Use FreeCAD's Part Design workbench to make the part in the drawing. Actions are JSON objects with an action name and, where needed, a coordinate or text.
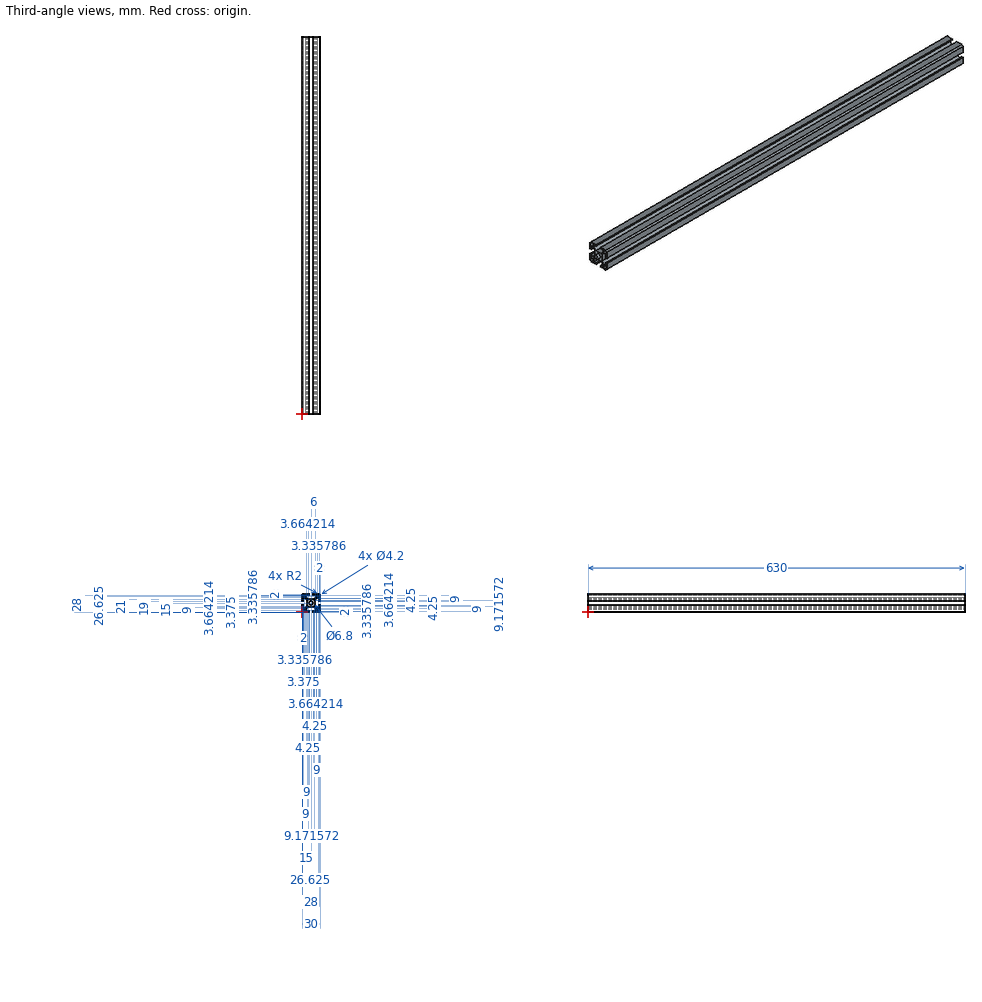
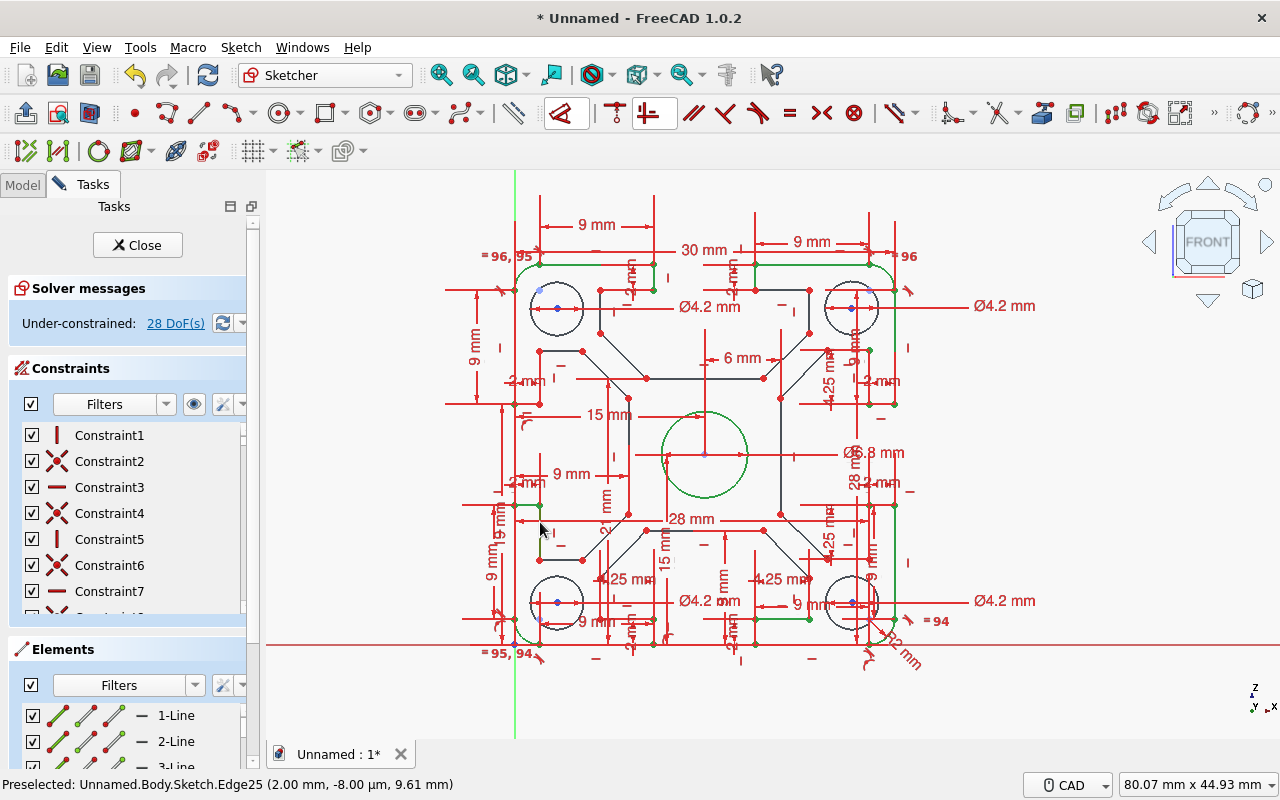
{"action": "left_click", "coordinate": [584, 114]}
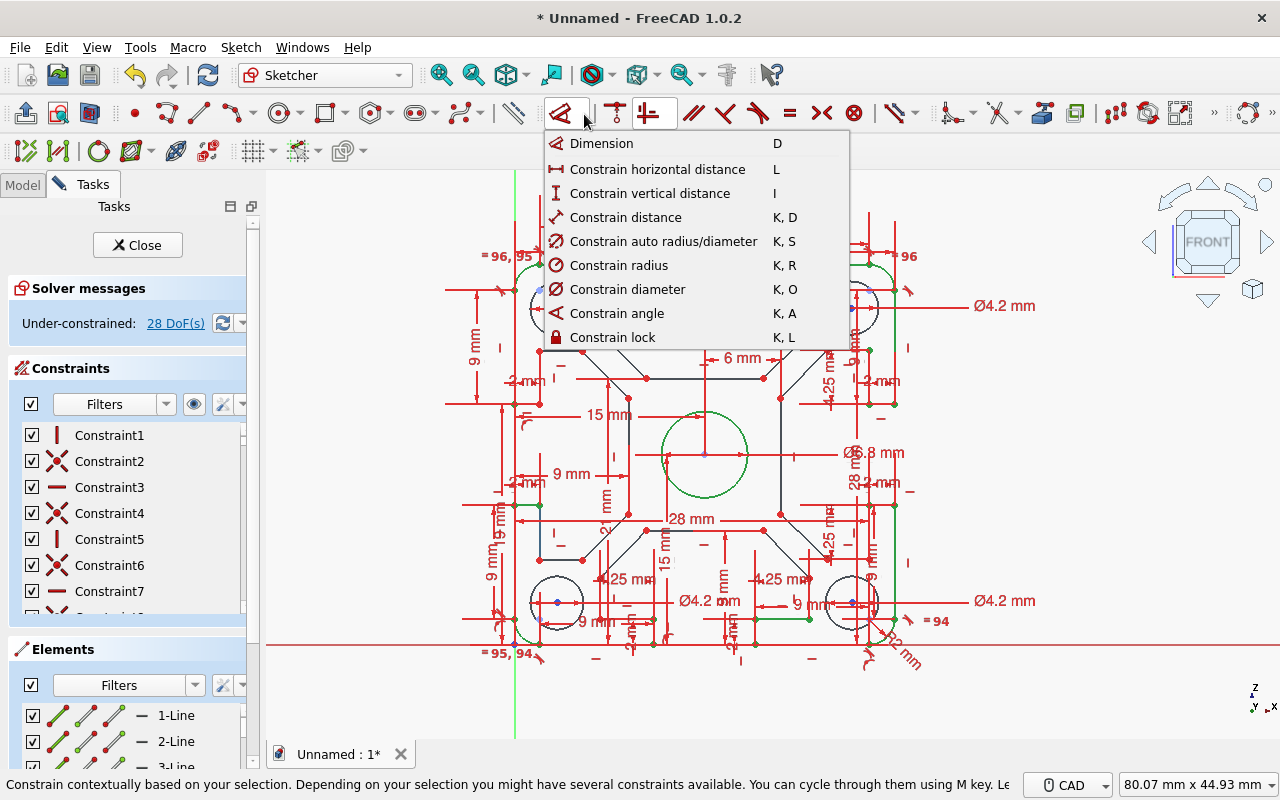
{"action": "left_click", "coordinate": [697, 193]}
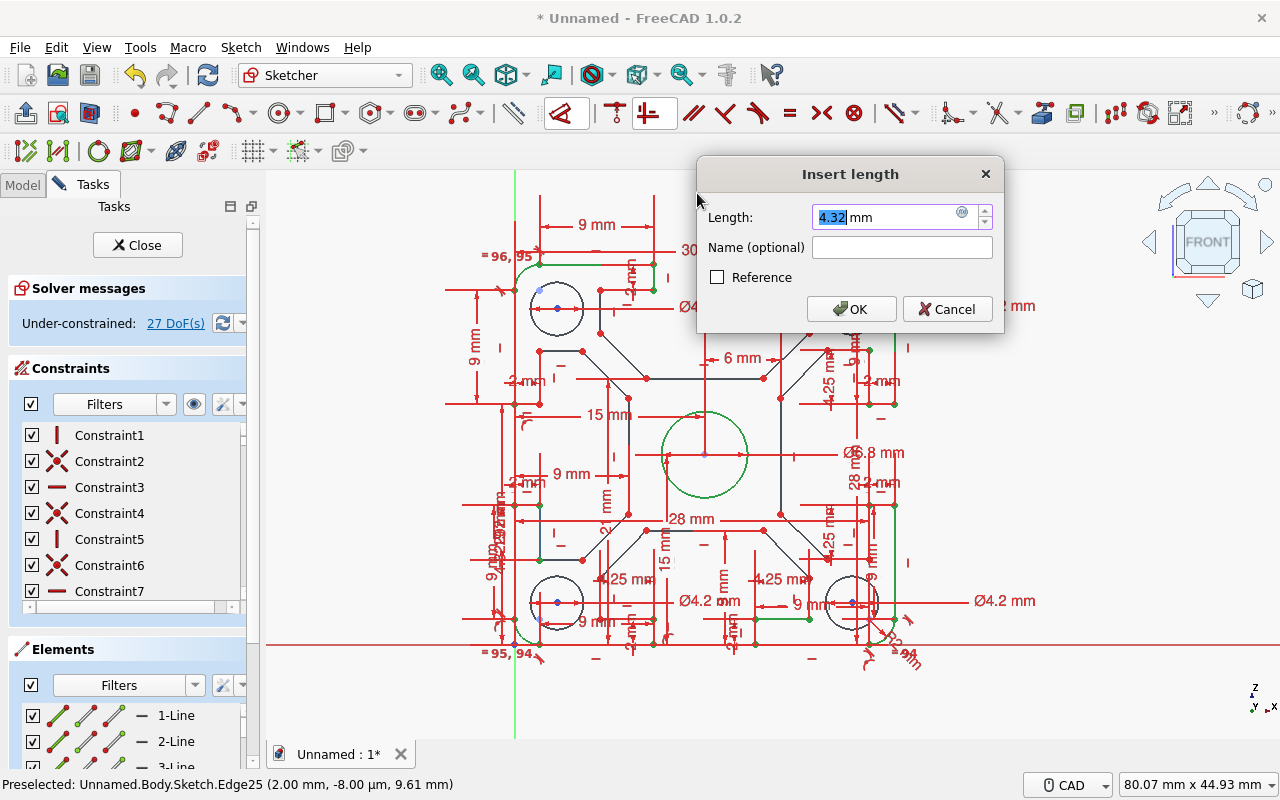
{"action": "type", "text": "4.25"}
{"action": "key", "text": "Return"}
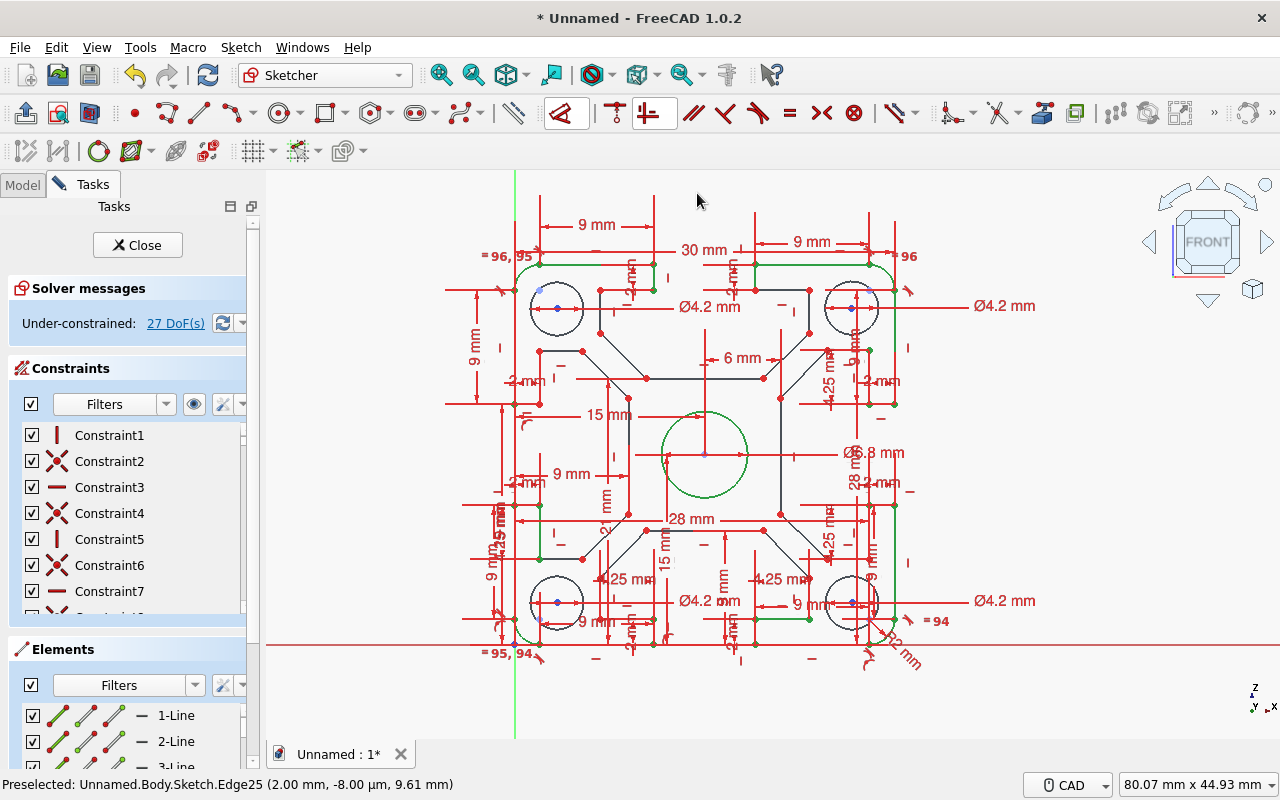
{"action": "left_click", "coordinate": [540, 367]}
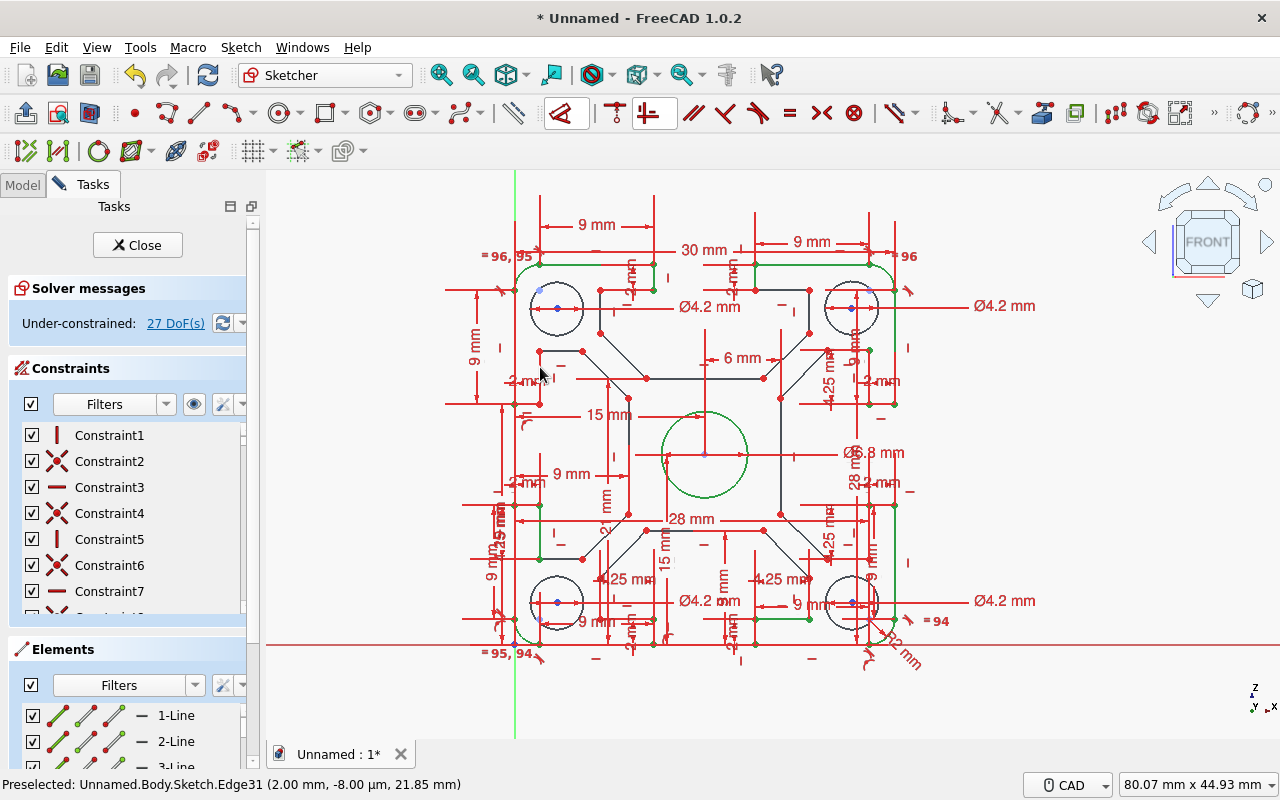
{"action": "key", "text": "i"}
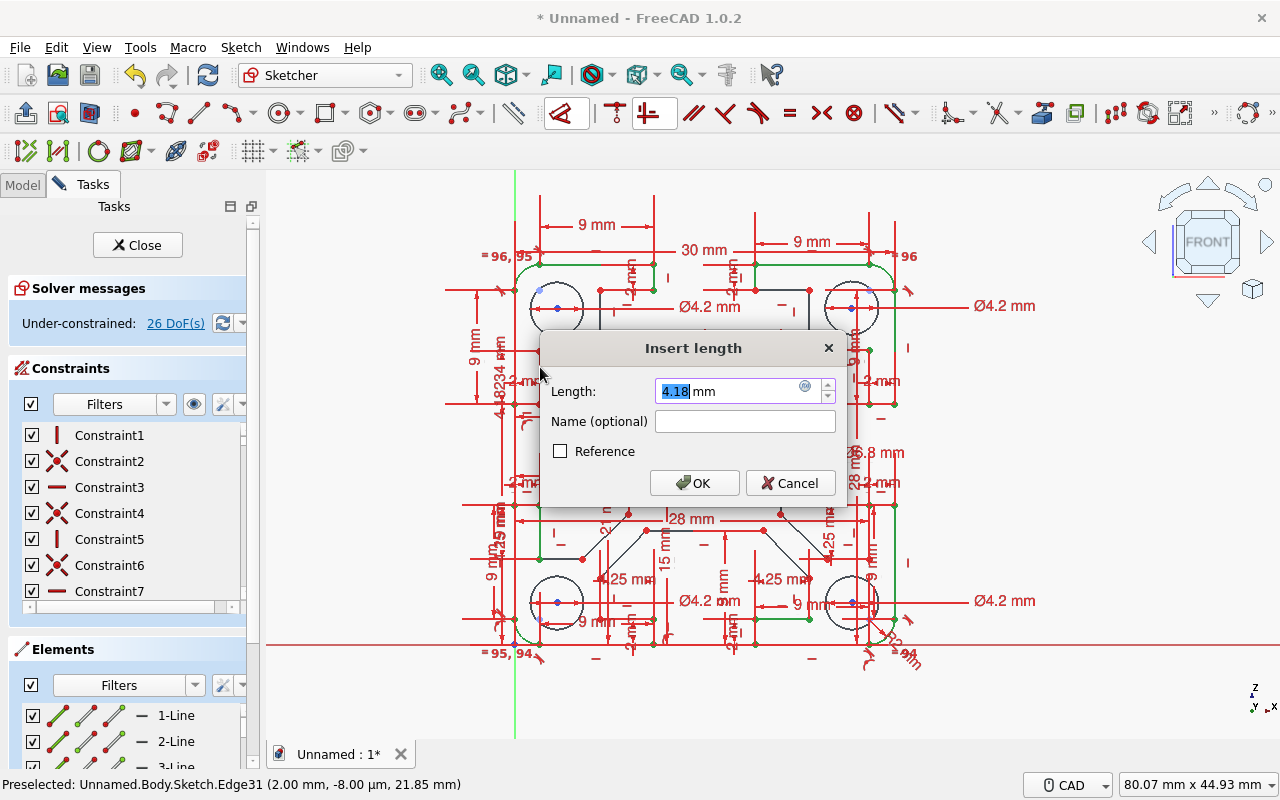
{"action": "type", "text": "4.25"}
{"action": "key", "text": "Return"}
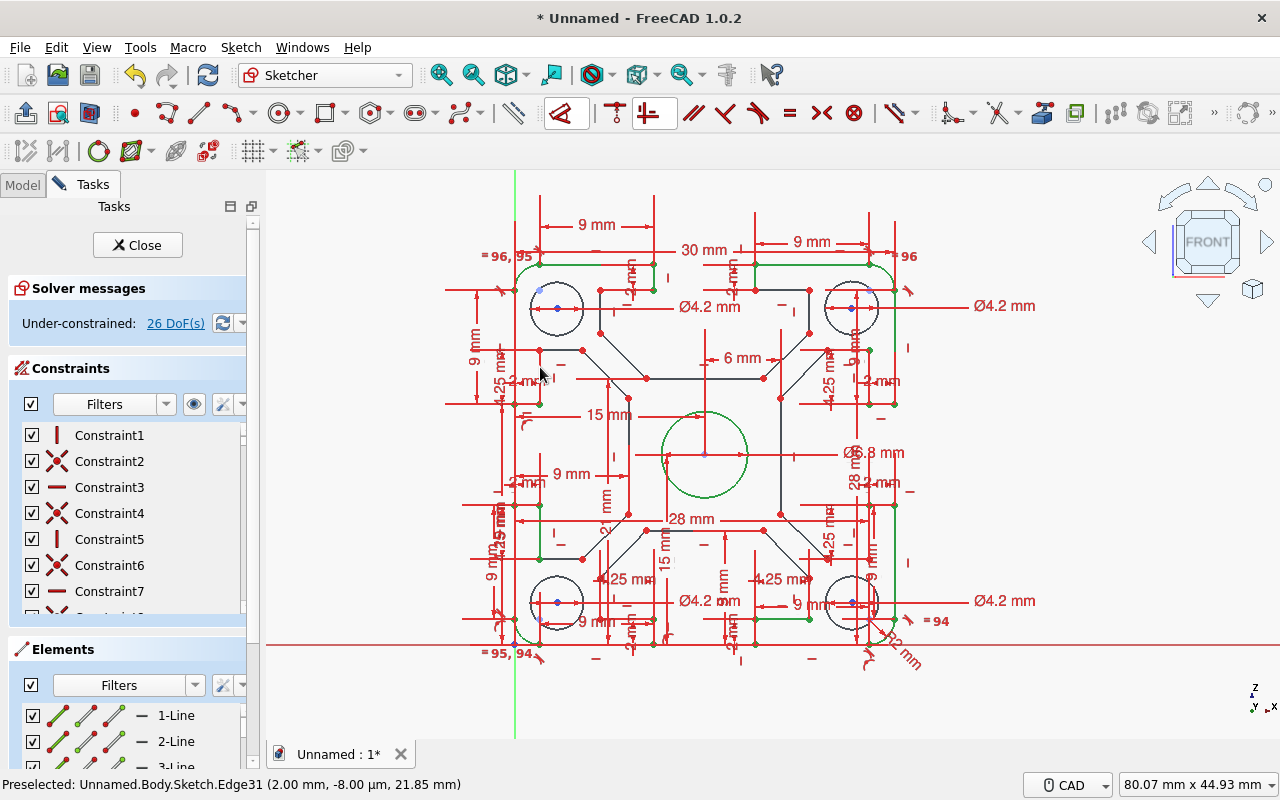
{"action": "left_click", "coordinate": [616, 290]}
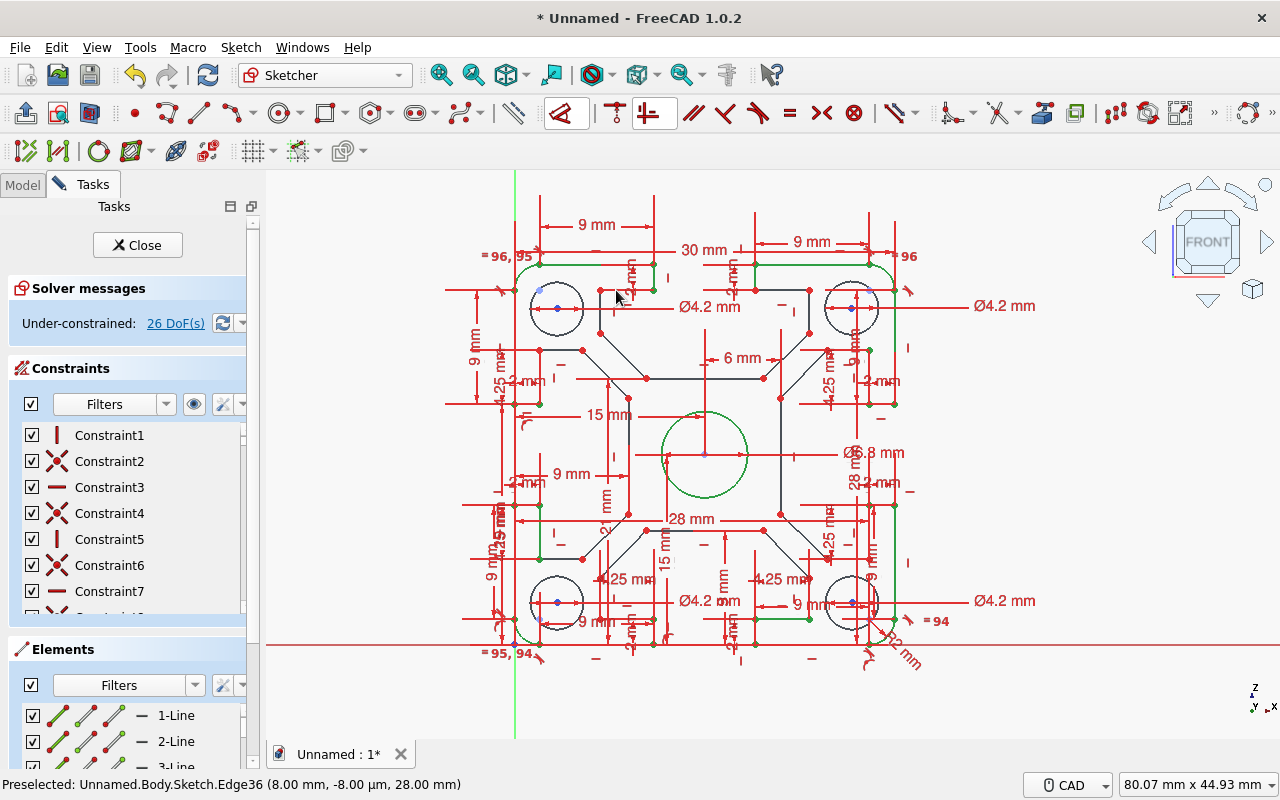
{"action": "left_click", "coordinate": [584, 114]}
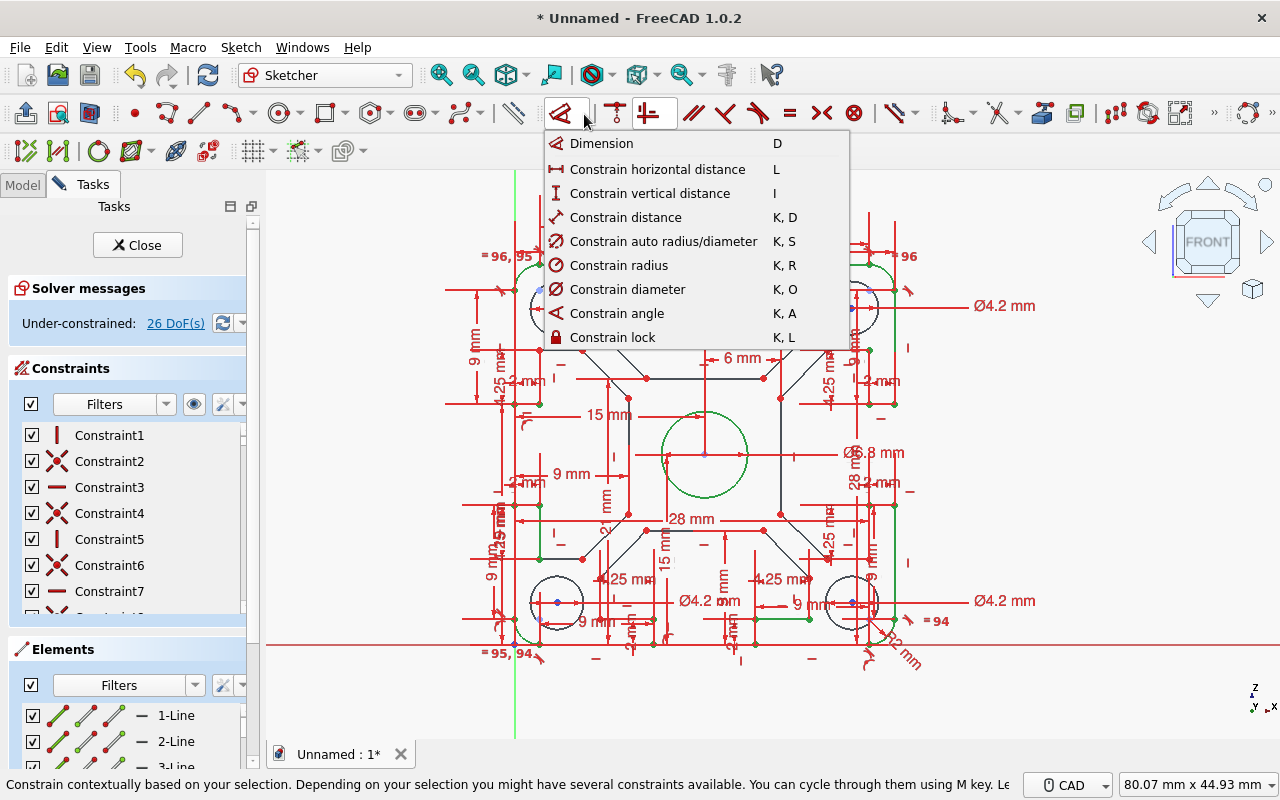
{"action": "left_click", "coordinate": [697, 169]}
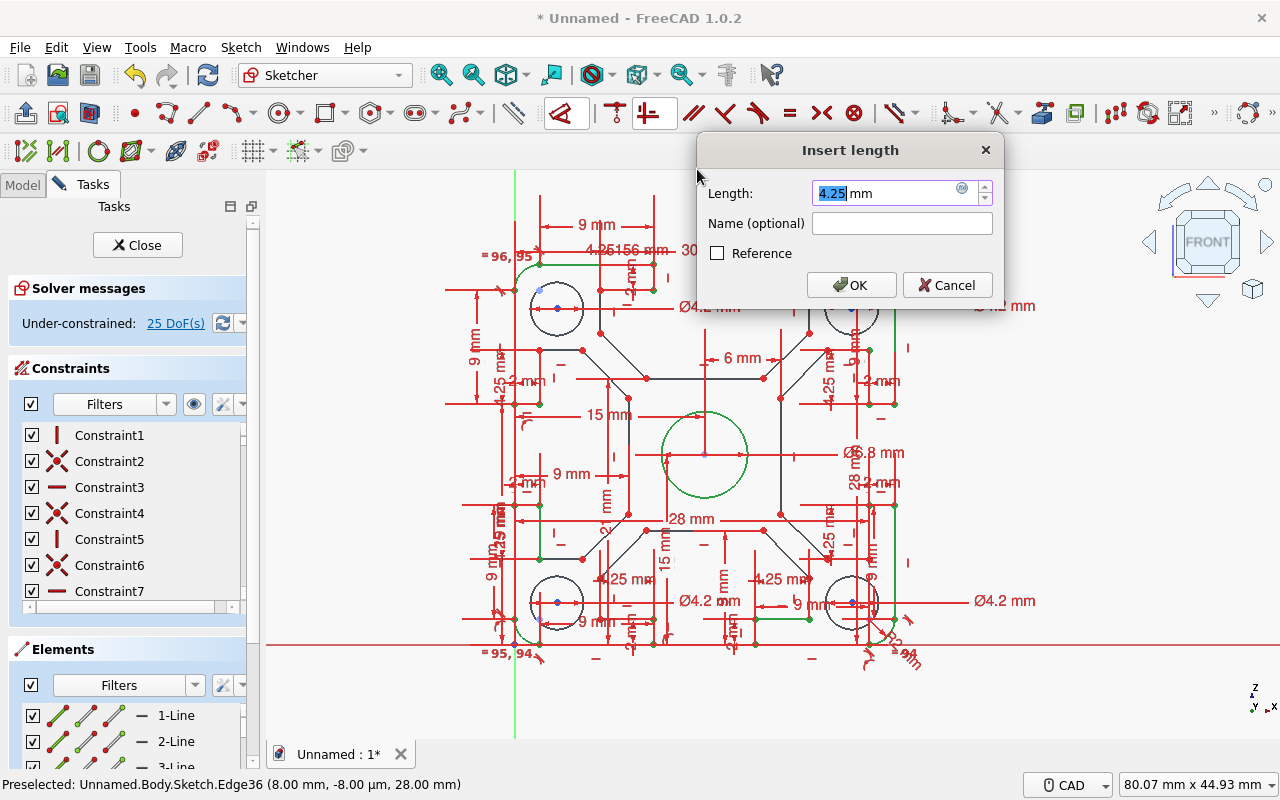
{"action": "type", "text": "4.25"}
{"action": "key", "text": "Return"}